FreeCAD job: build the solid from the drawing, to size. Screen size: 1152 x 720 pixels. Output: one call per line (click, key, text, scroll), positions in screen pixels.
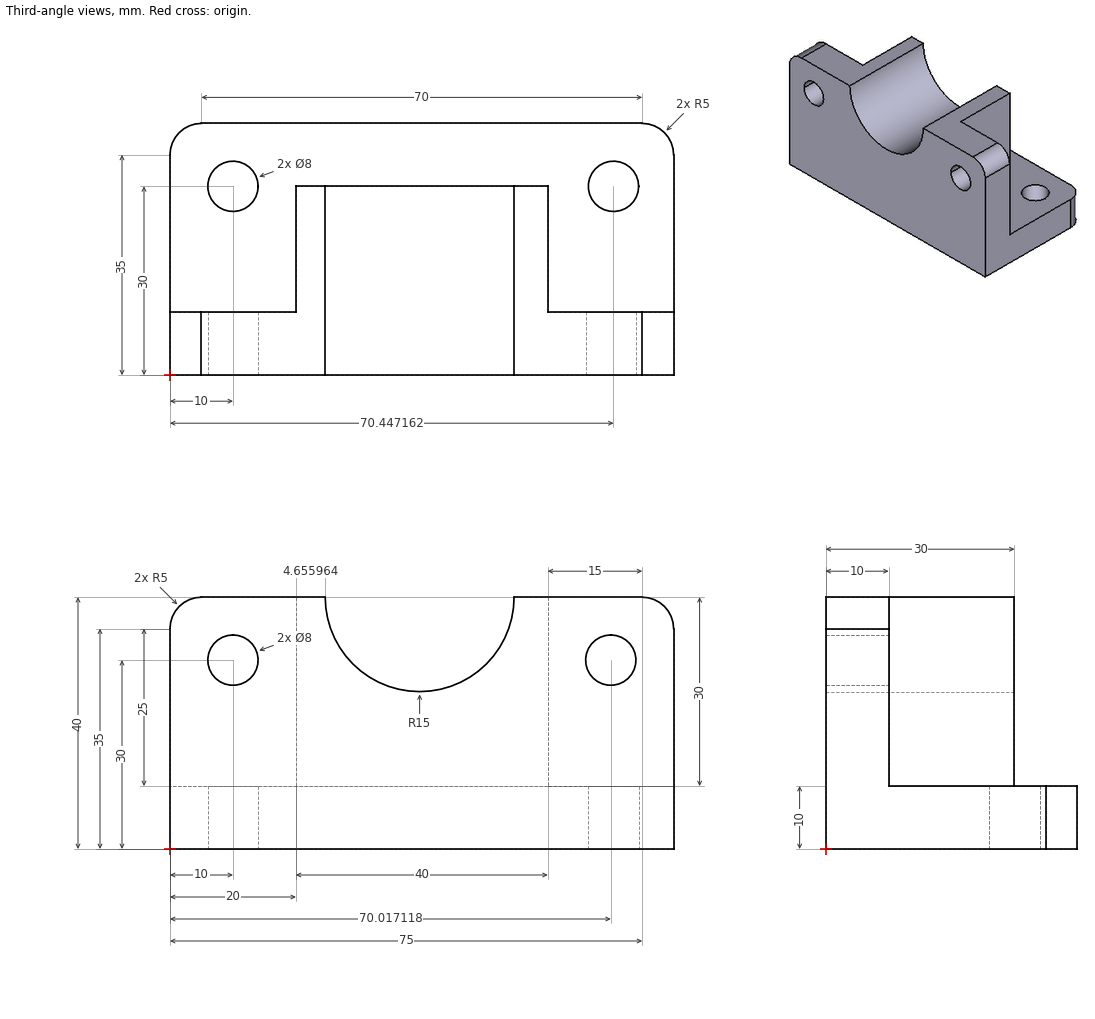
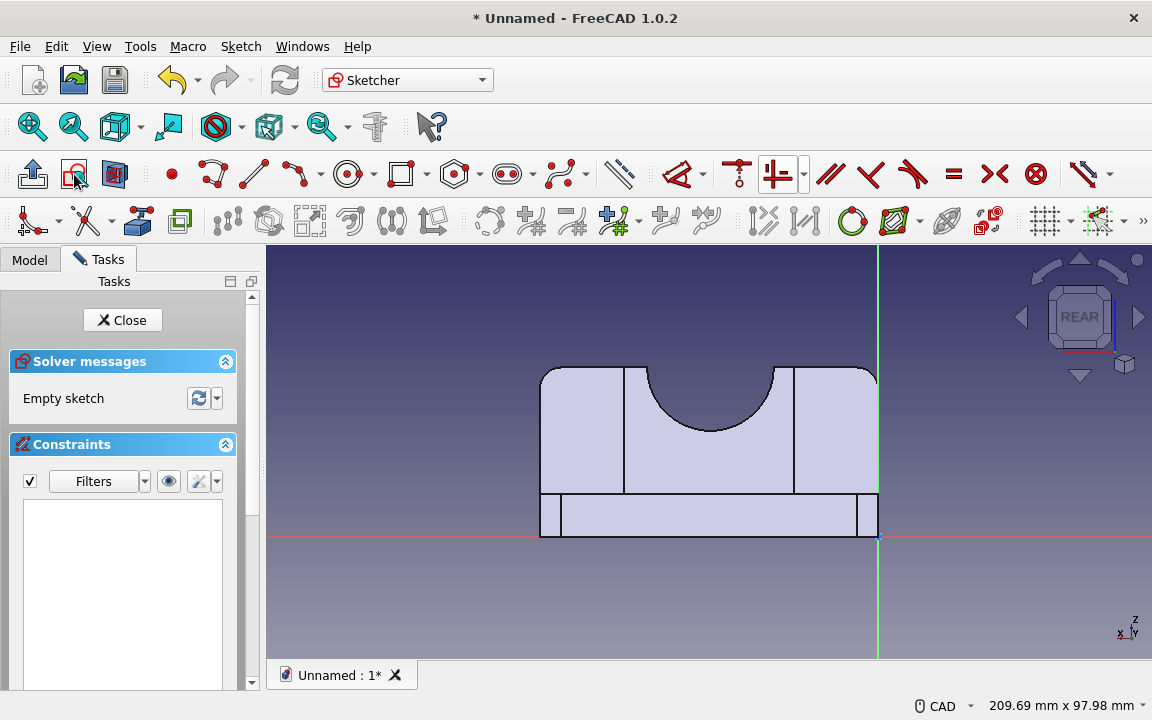
click(115, 174)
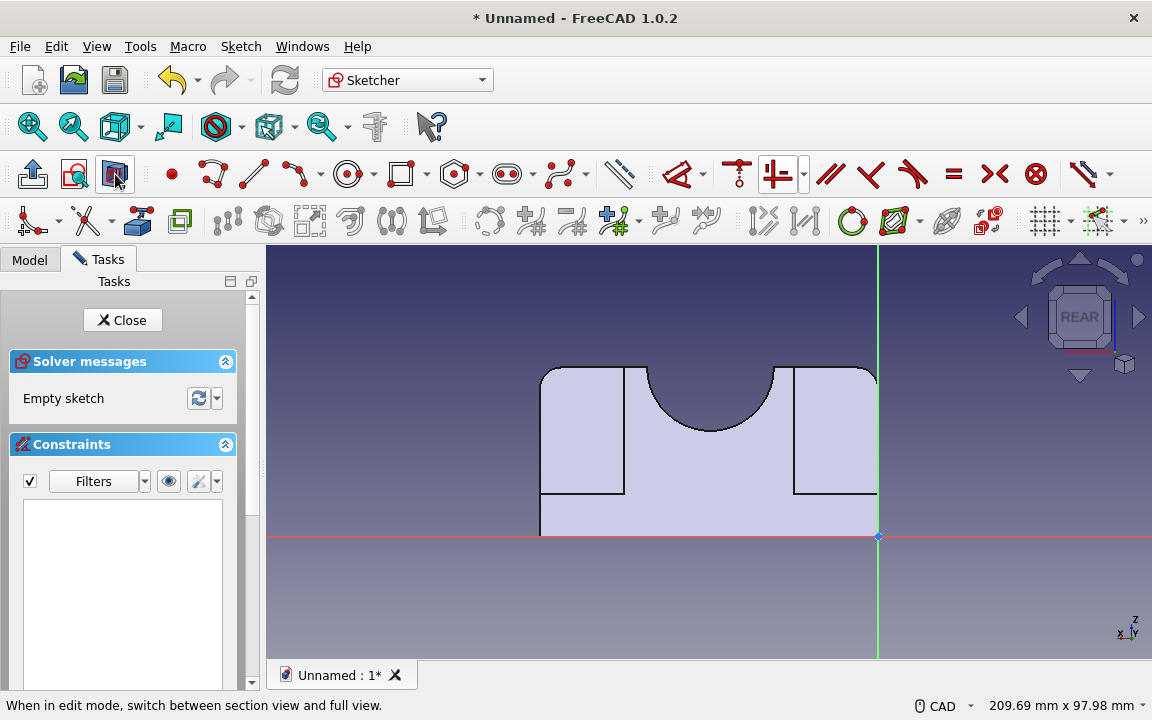
scroll(887, 490, up, 2)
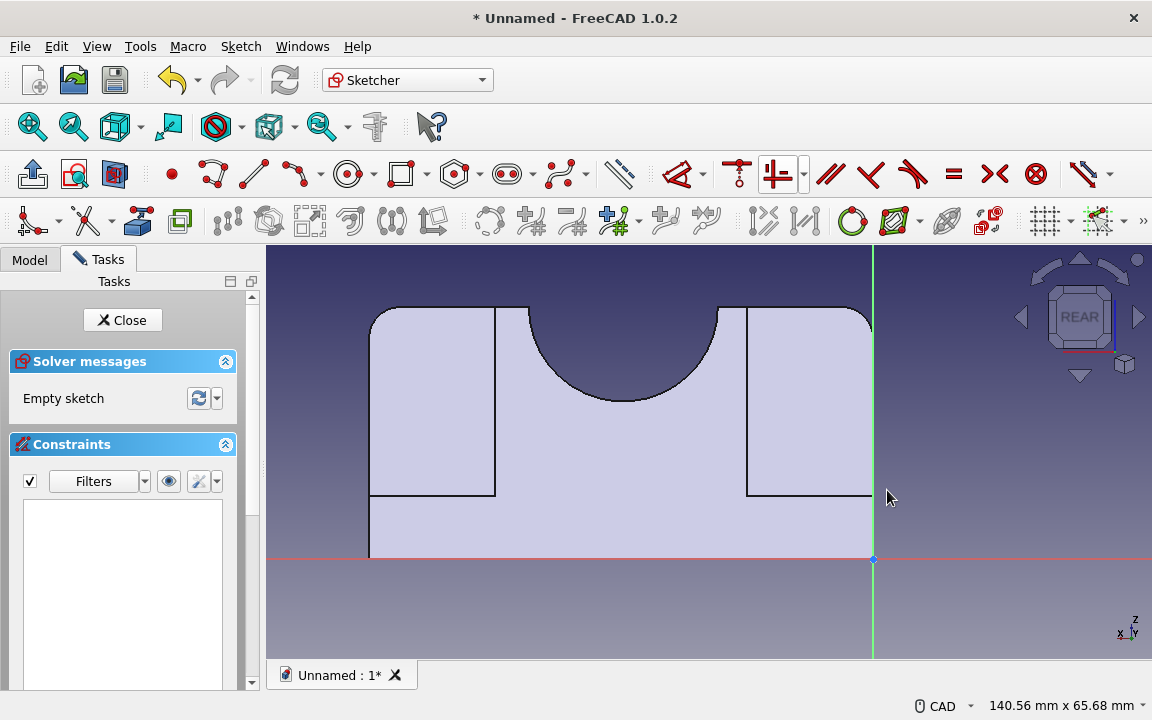
click(348, 174)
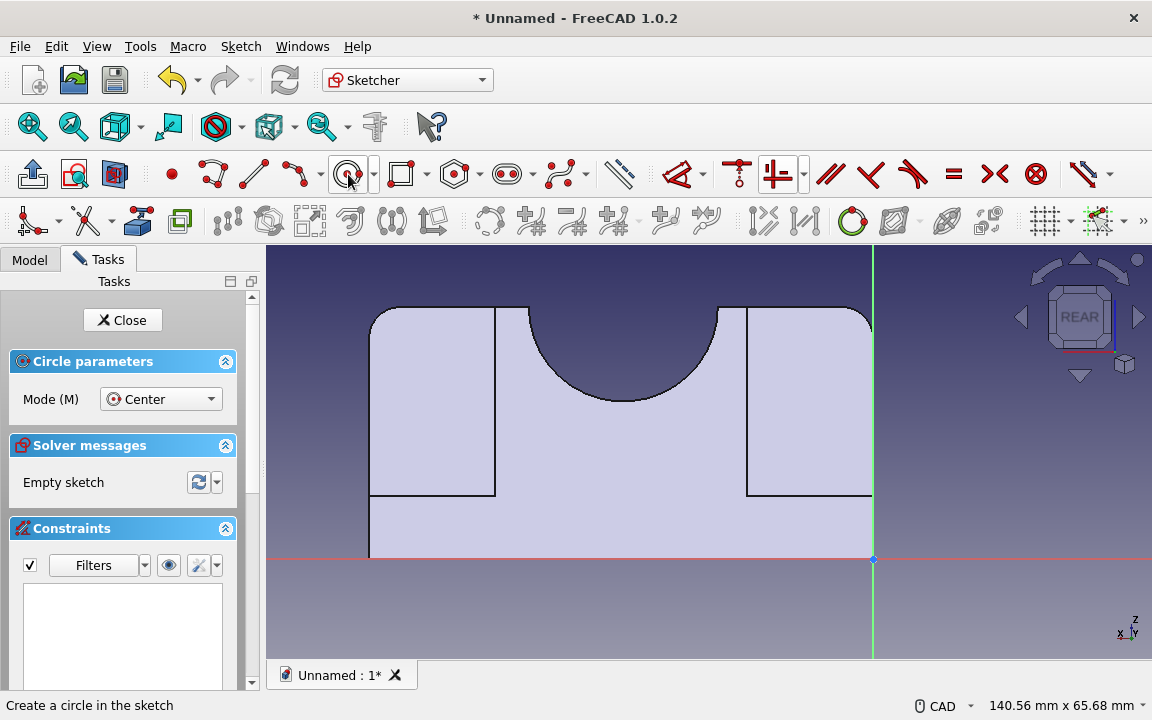
click(810, 370)
click(828, 352)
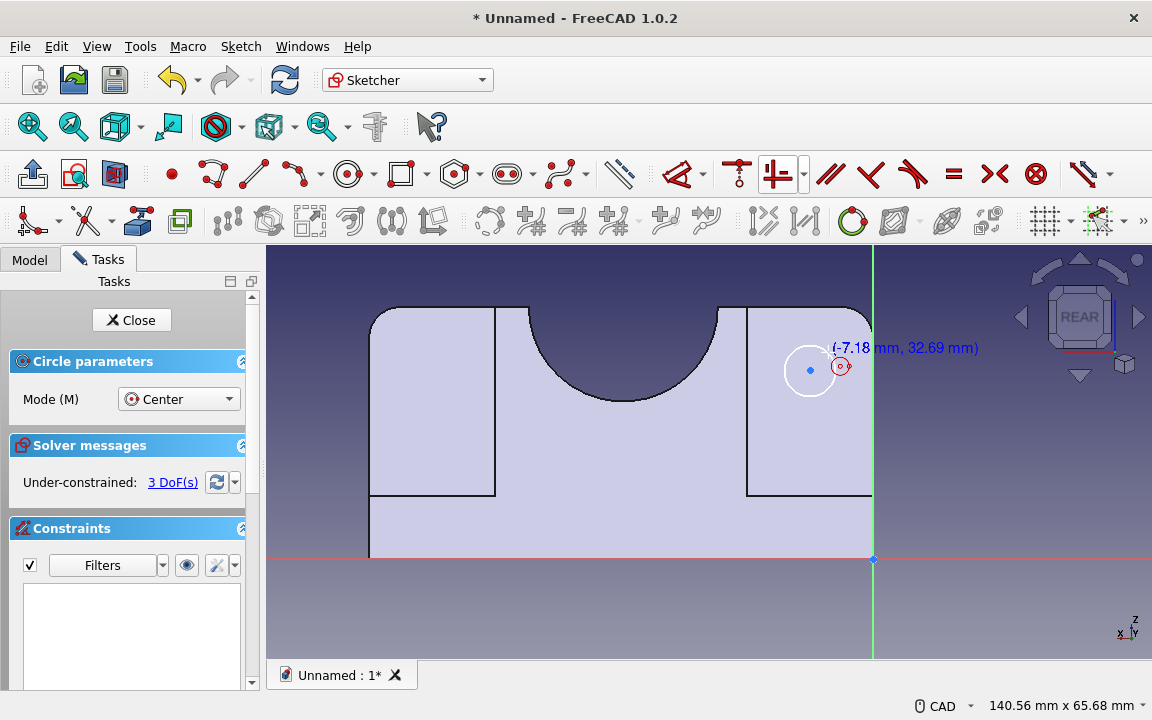
click(432, 370)
click(450, 352)
key(Escape)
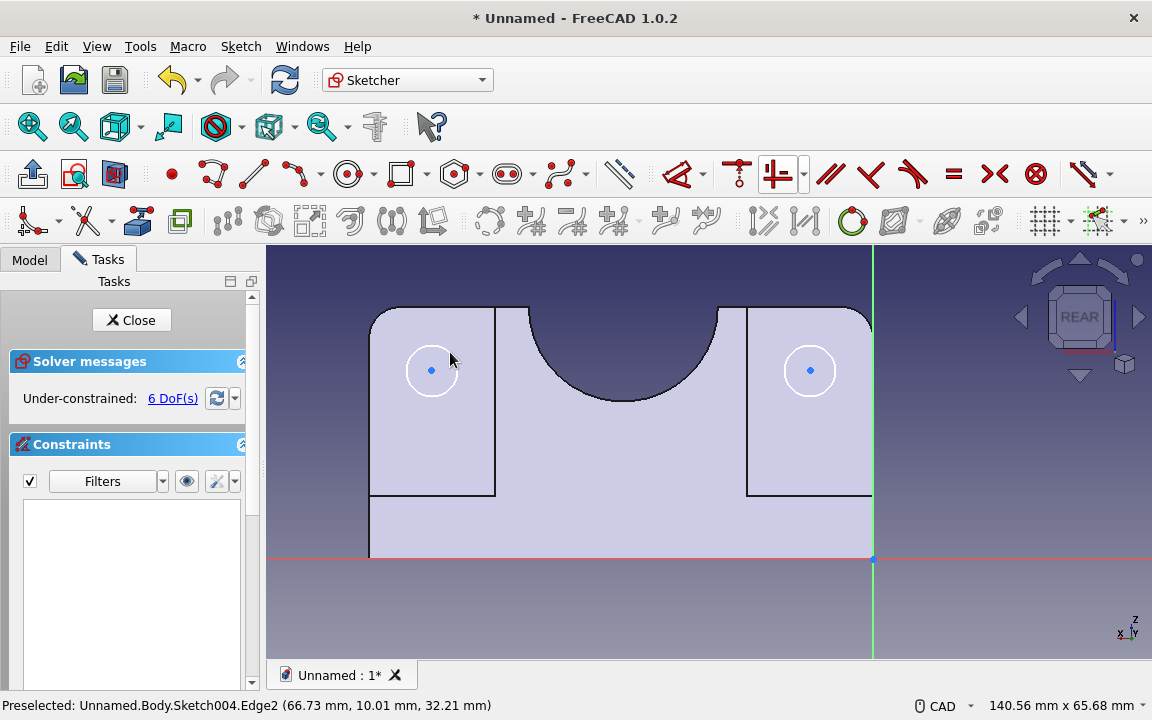
click(828, 353)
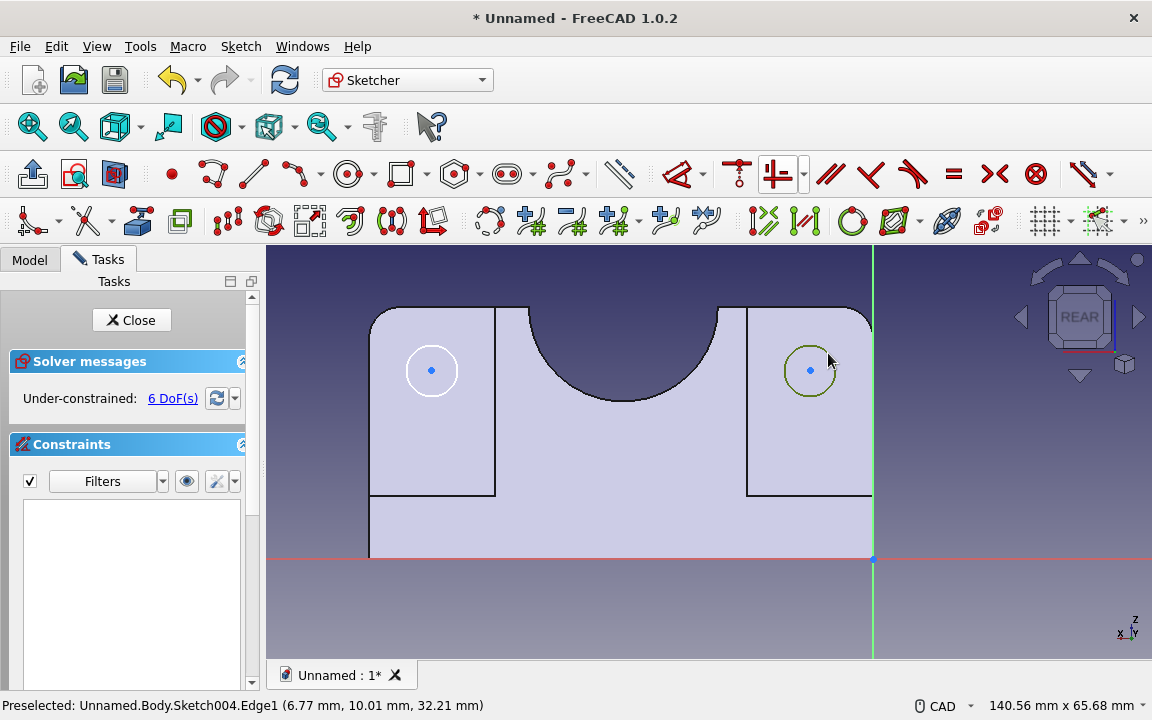
click(450, 353)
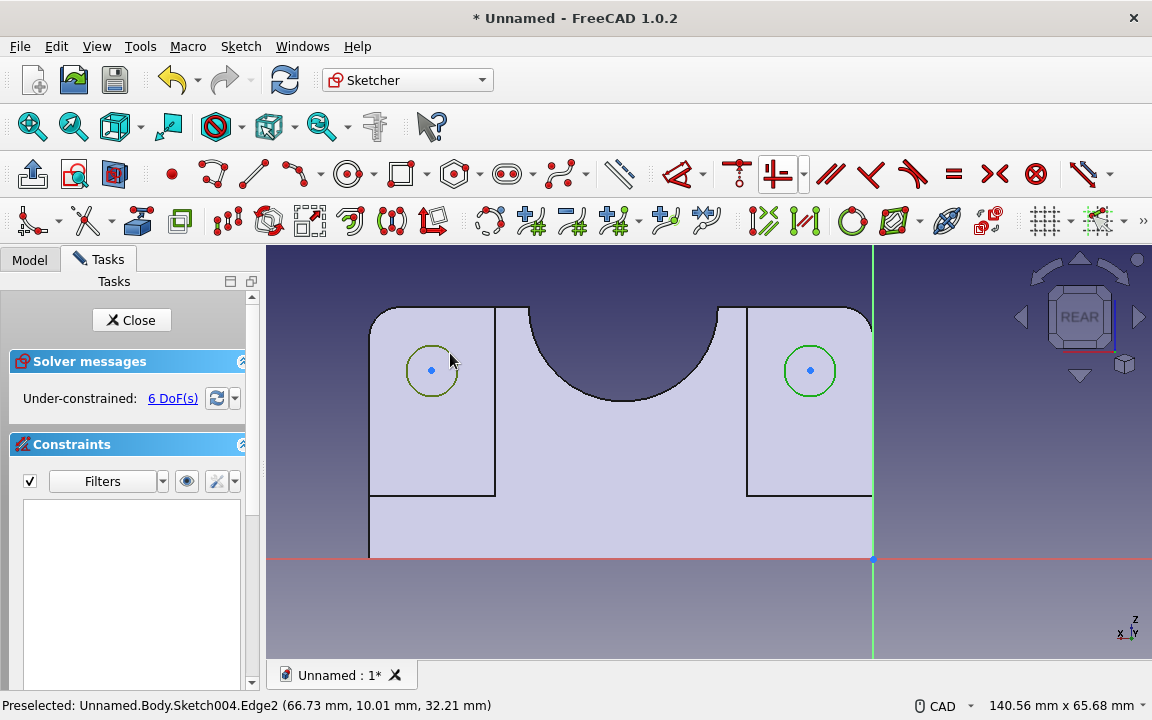
click(954, 174)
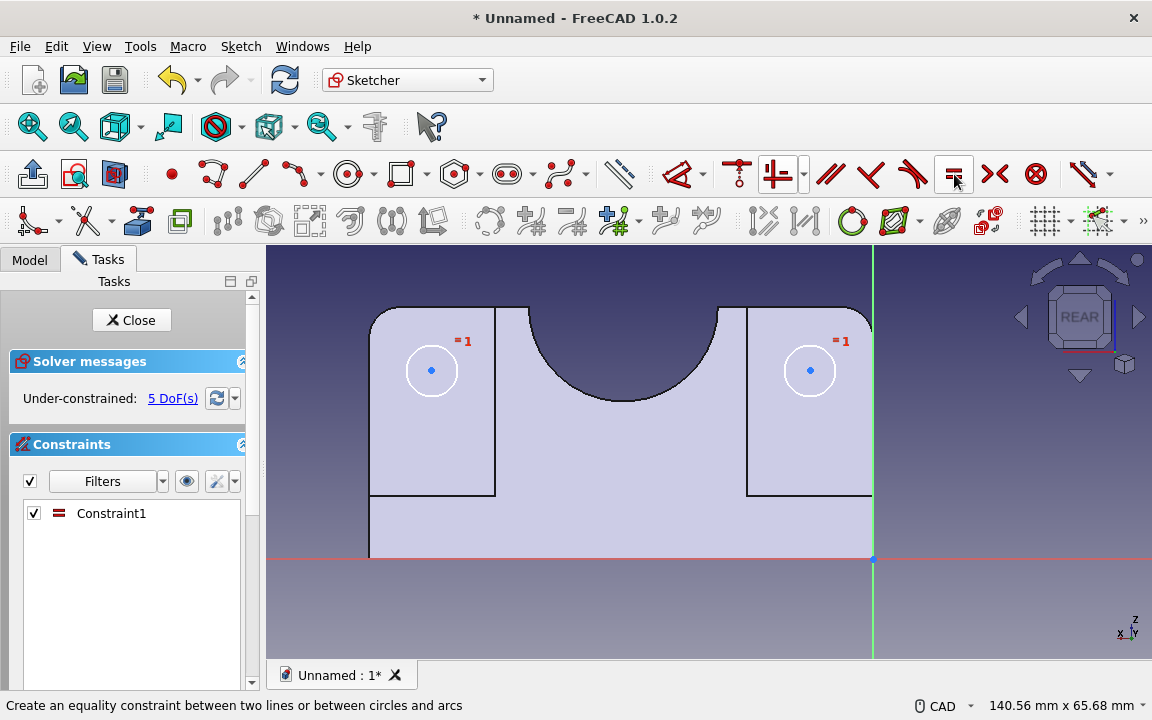
click(810, 371)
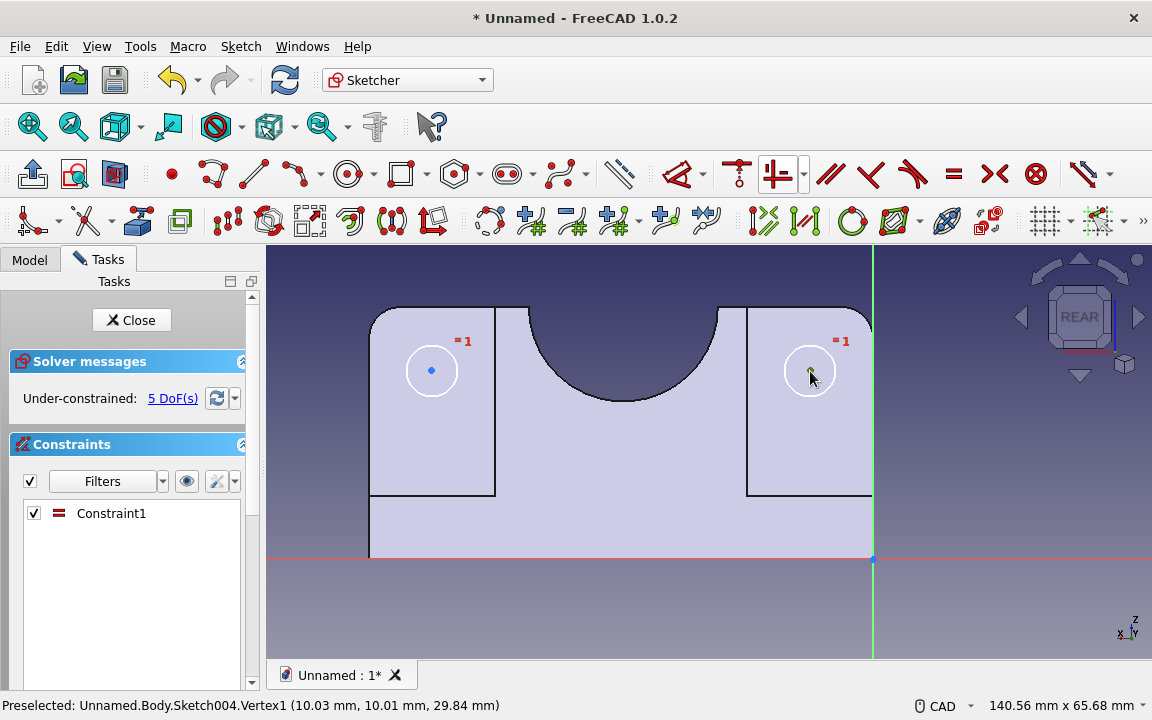
click(432, 371)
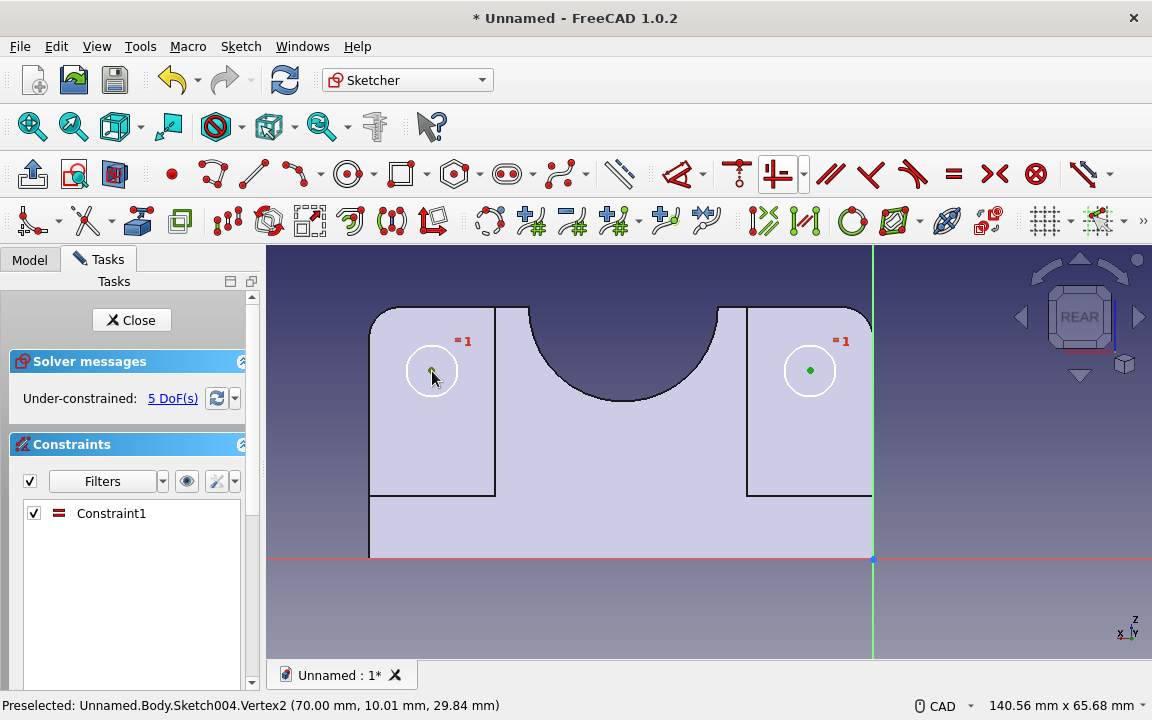
key(h)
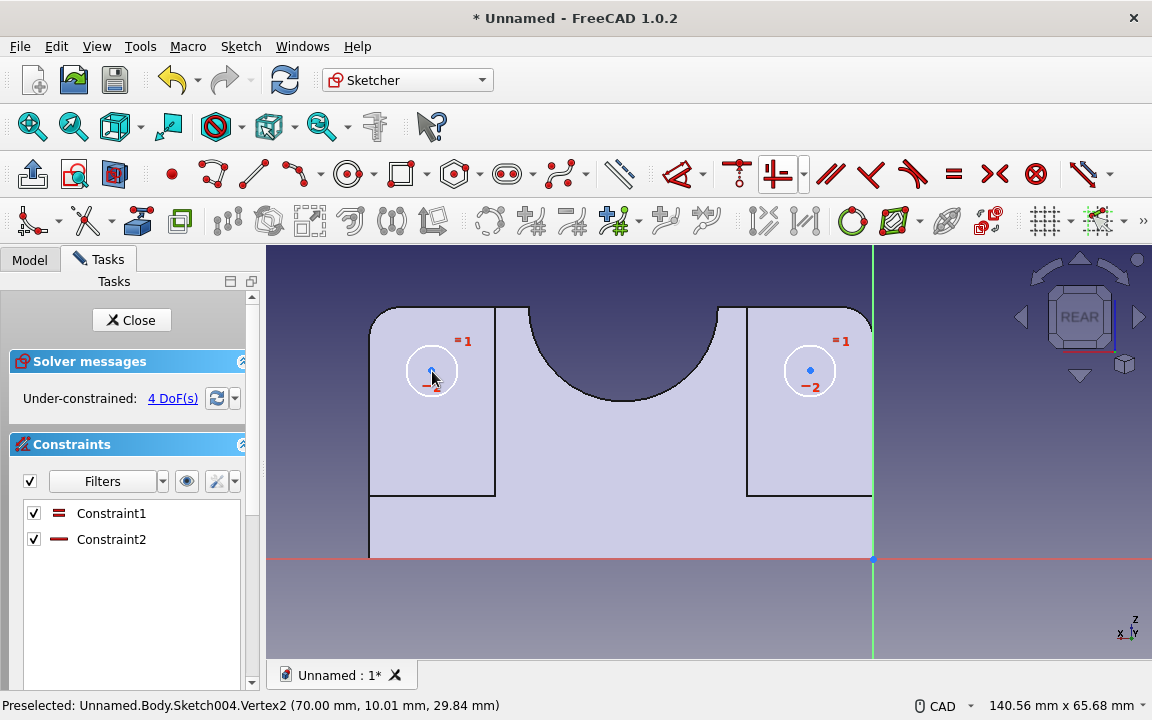
click(676, 174)